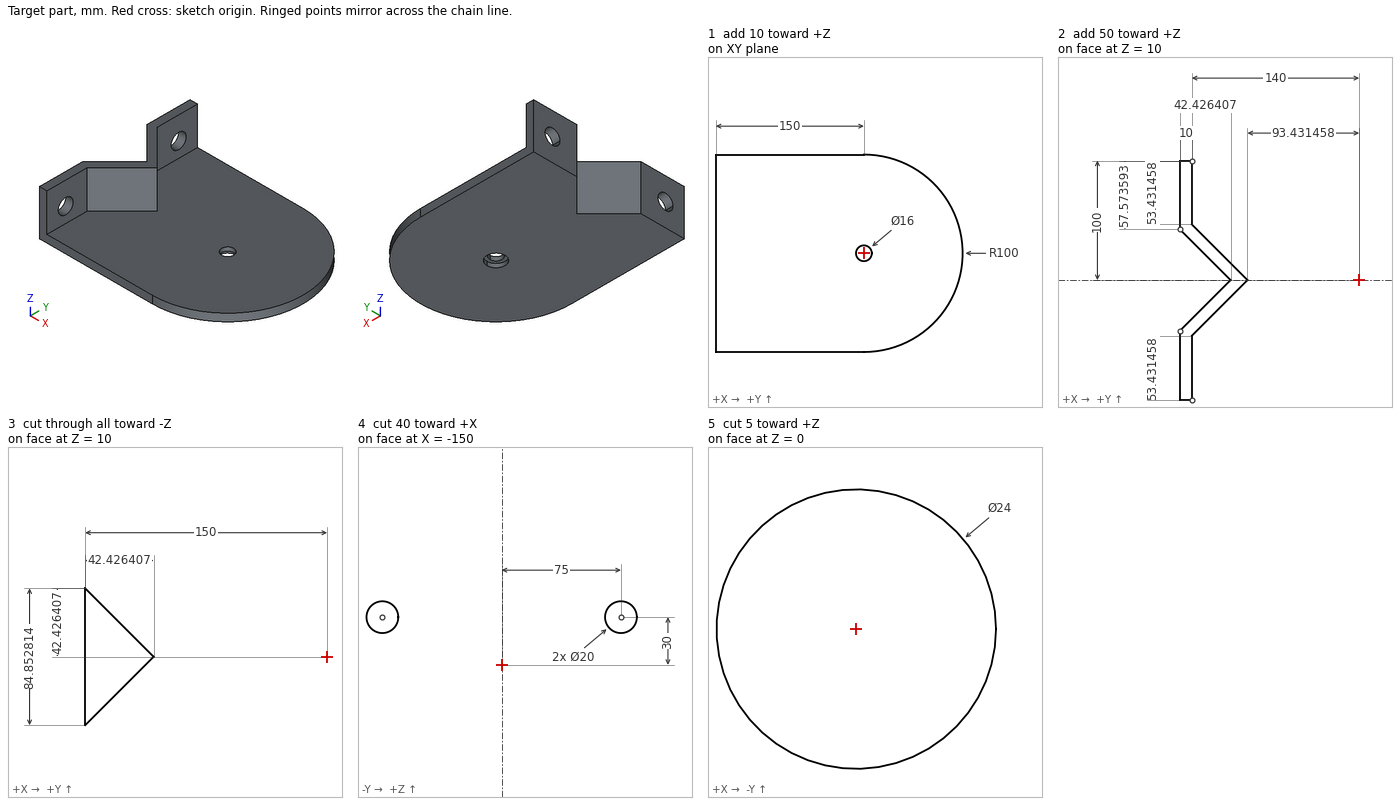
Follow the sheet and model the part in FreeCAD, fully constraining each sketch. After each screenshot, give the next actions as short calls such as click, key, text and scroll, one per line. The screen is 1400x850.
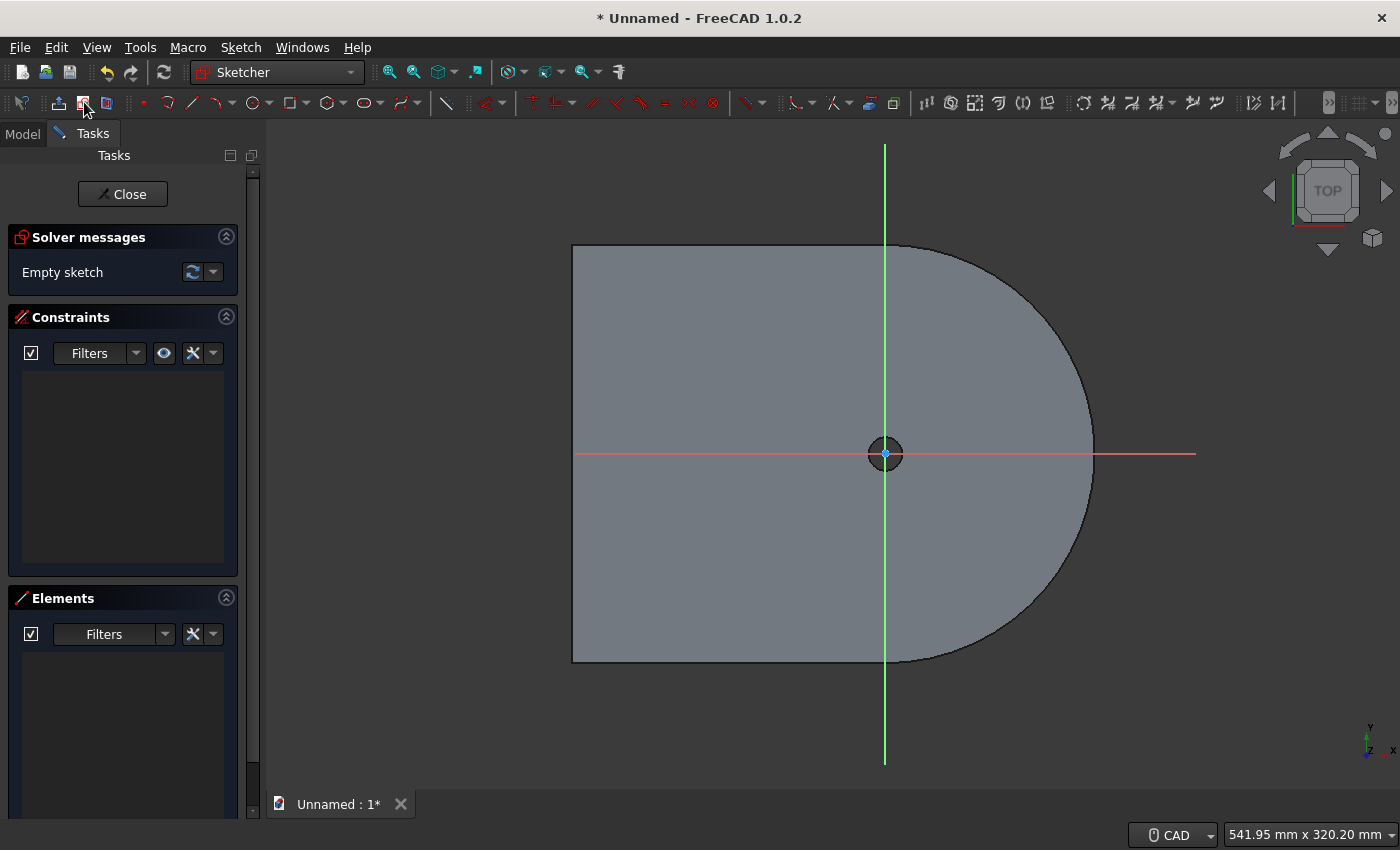
click(690, 454)
click(593, 357)
click(593, 245)
click(572, 245)
click(572, 365)
click(660, 454)
click(572, 543)
click(572, 663)
click(593, 663)
click(593, 551)
click(690, 454)
key(Escape)
key(Escape)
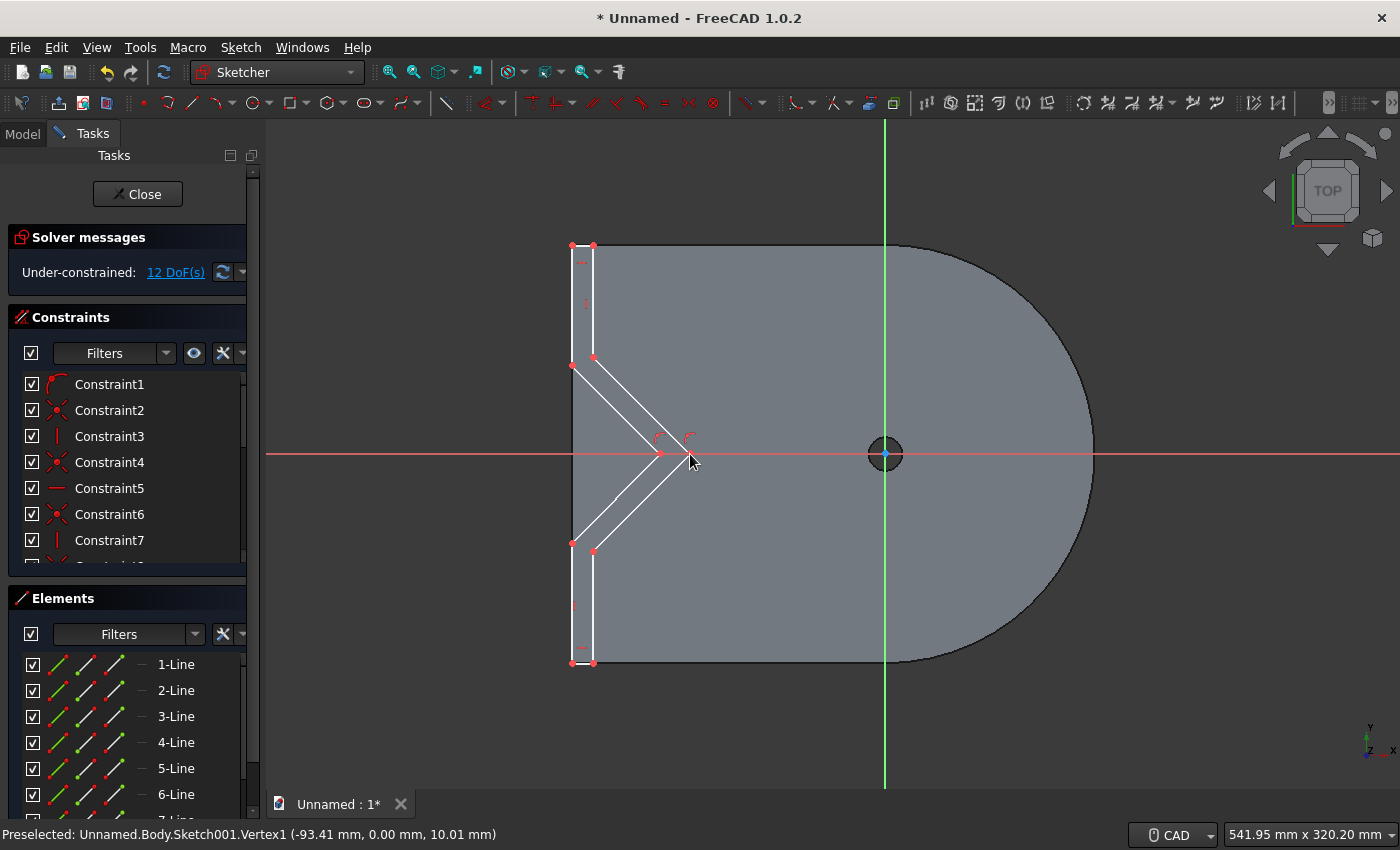
click(572, 366)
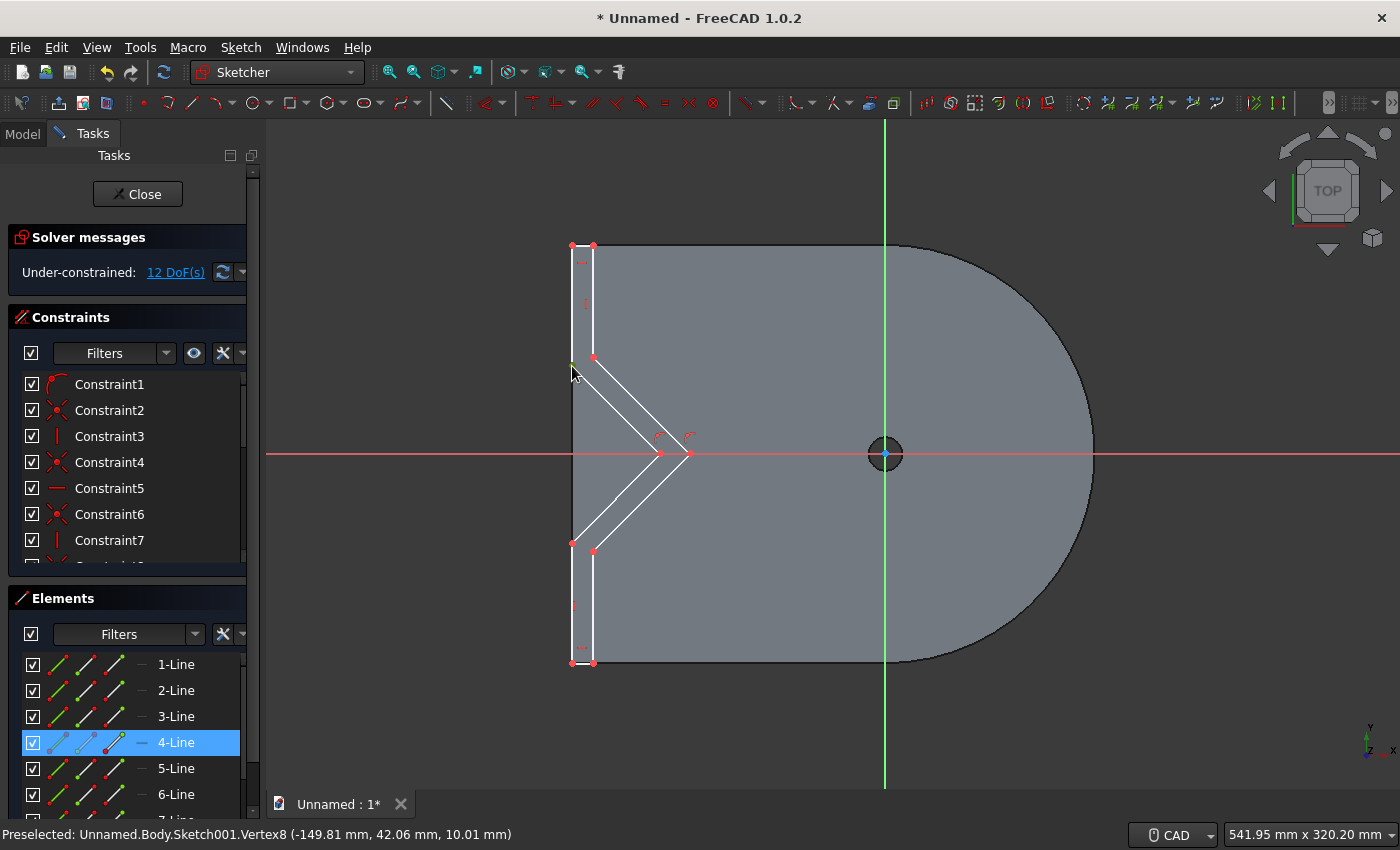
click(572, 544)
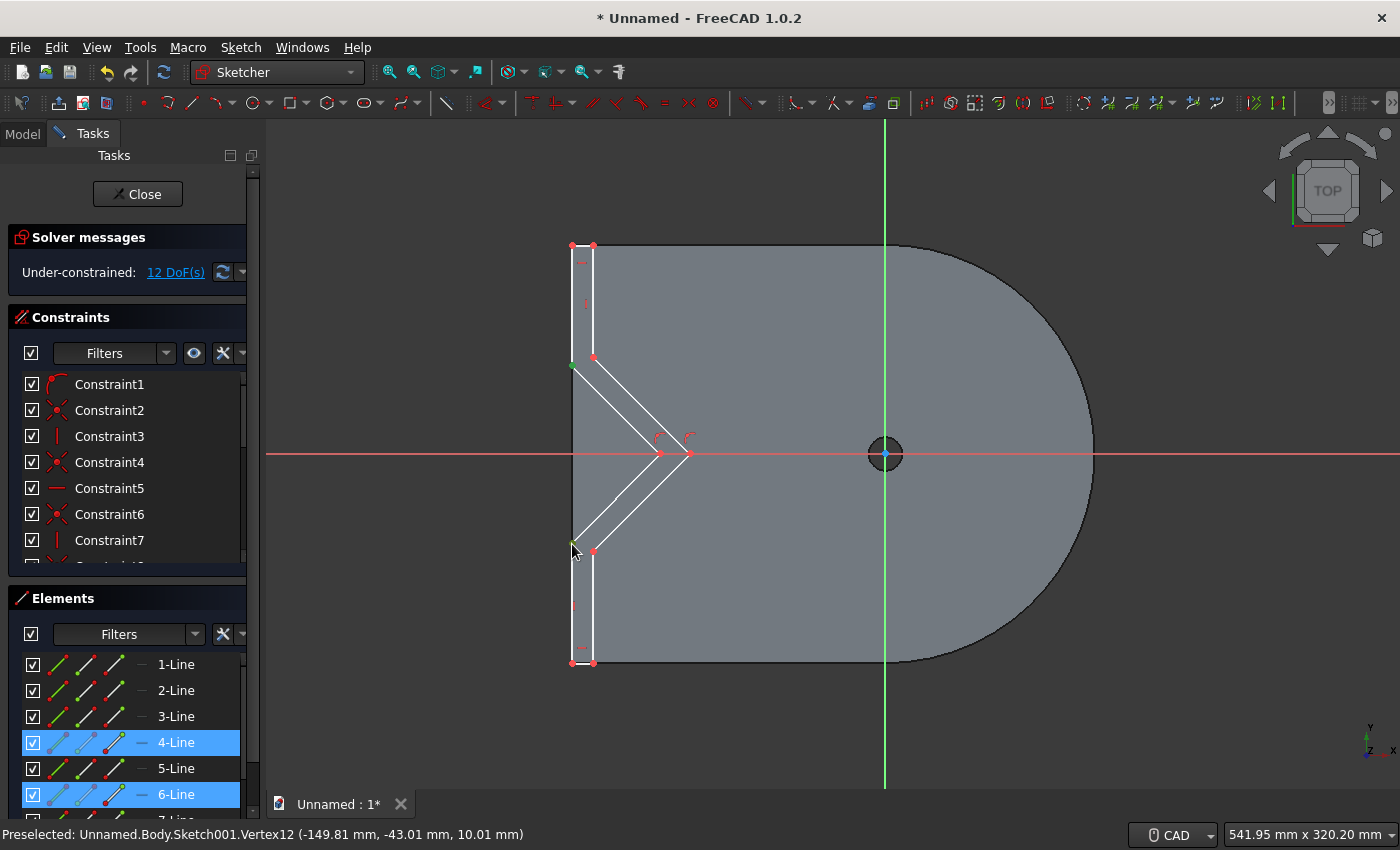
click(361, 454)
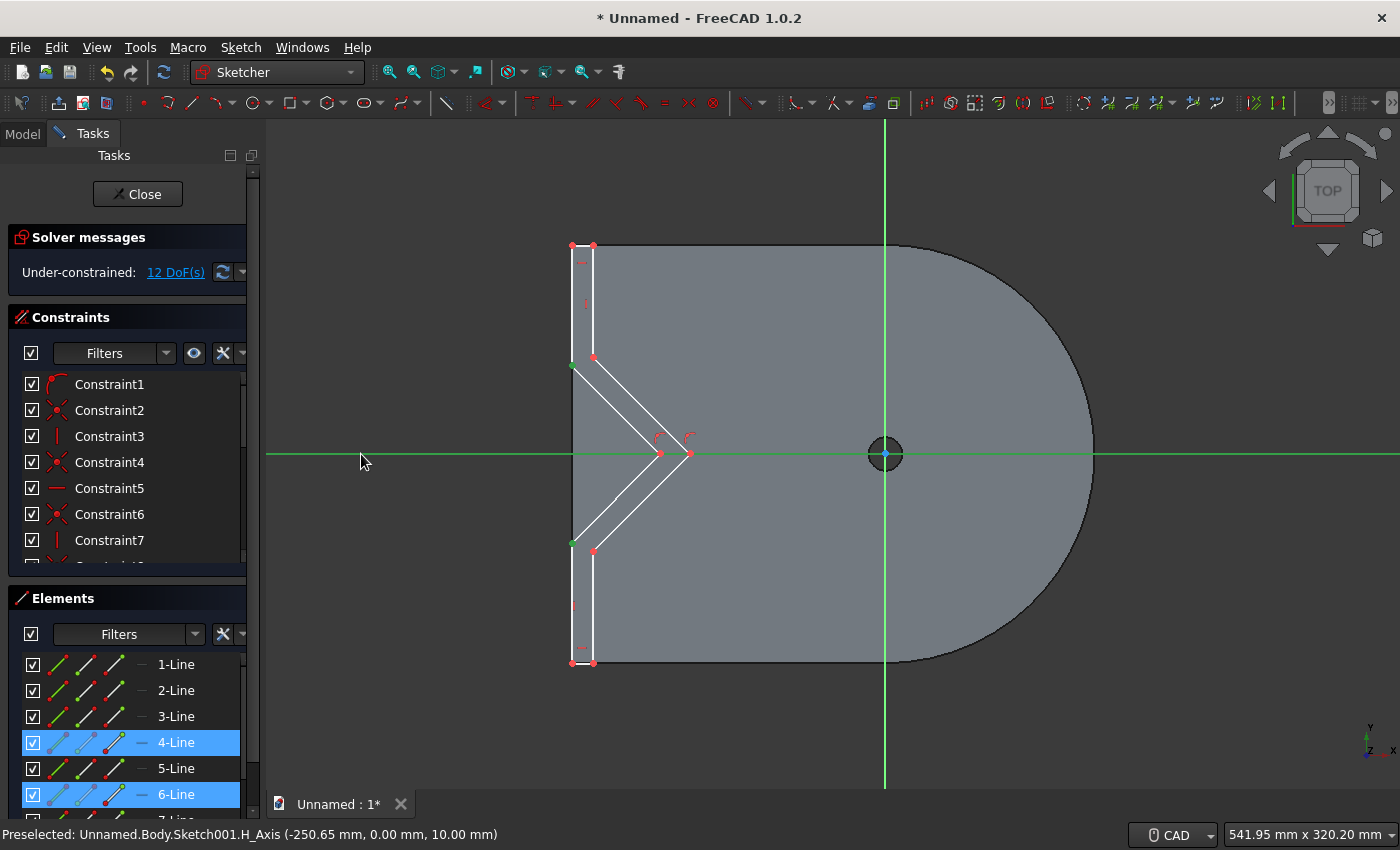
key(s)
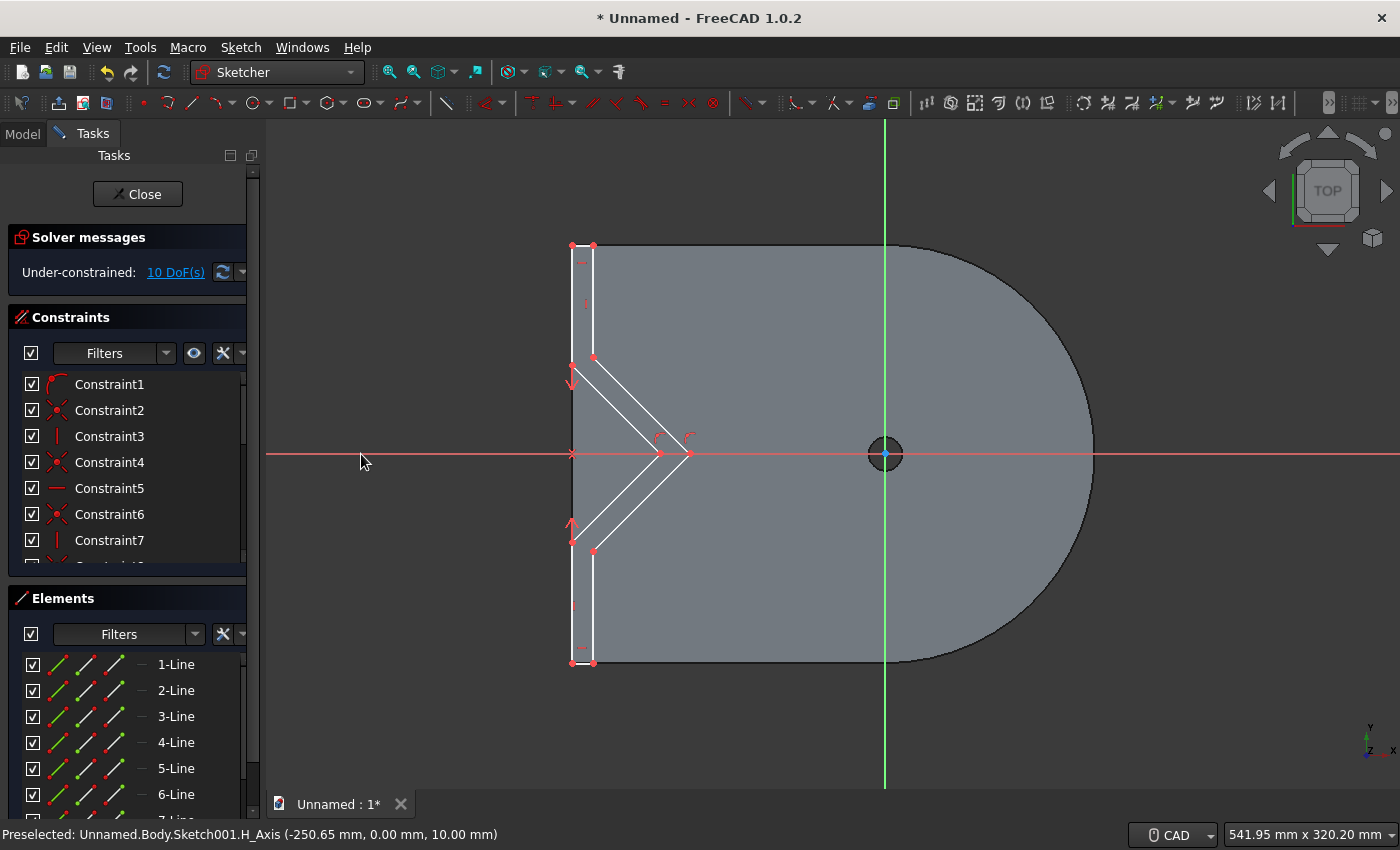
click(593, 246)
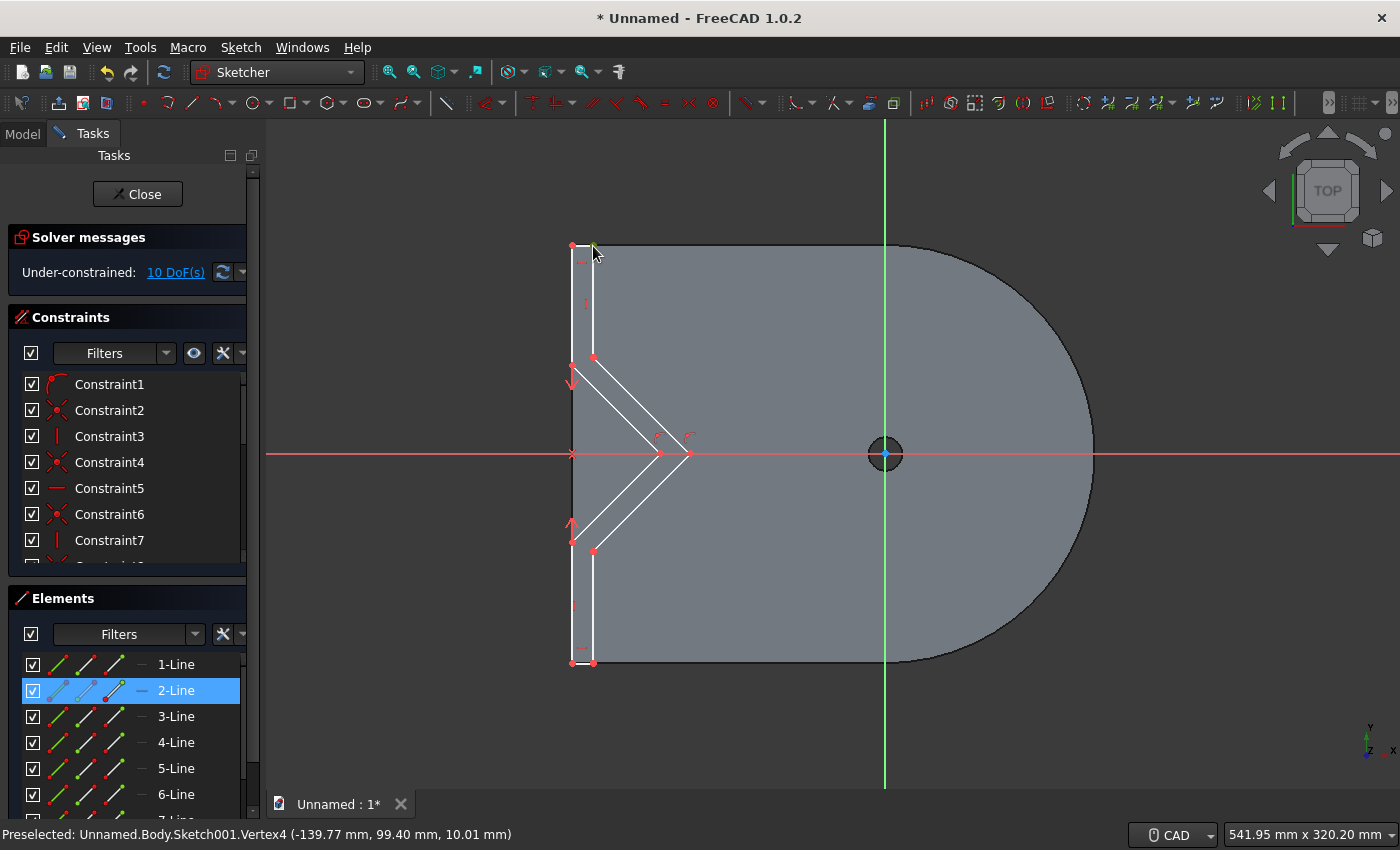
click(593, 664)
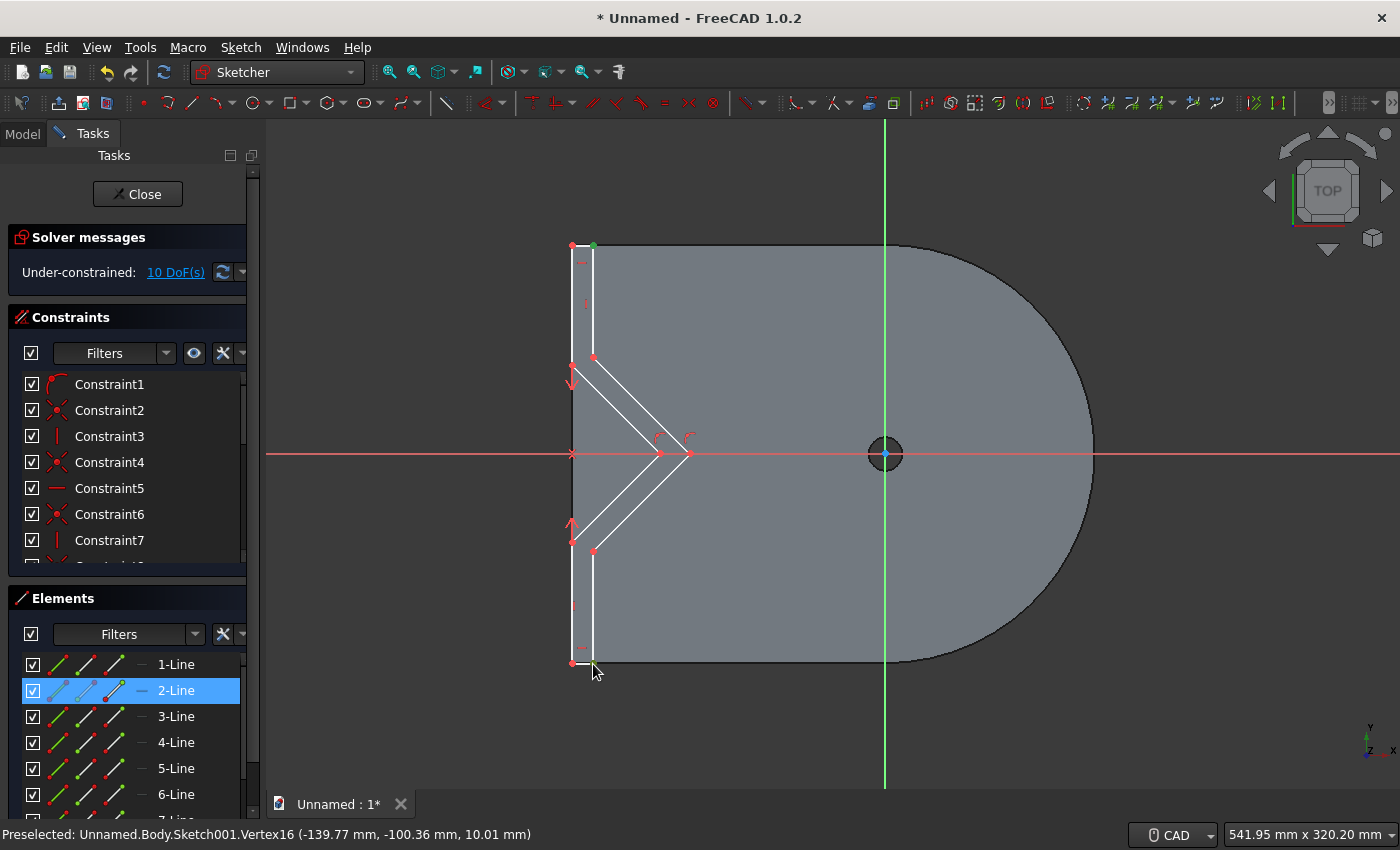
click(361, 454)